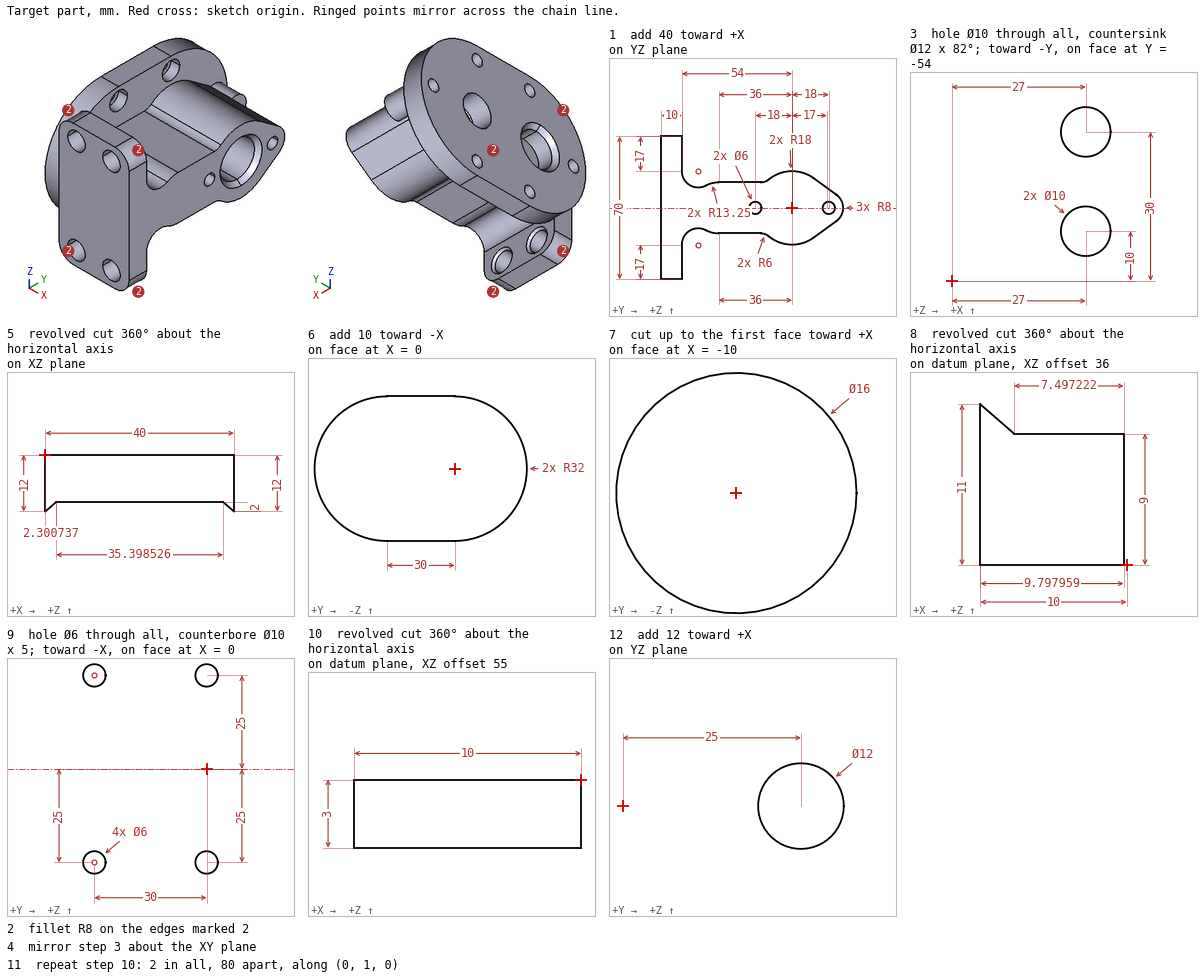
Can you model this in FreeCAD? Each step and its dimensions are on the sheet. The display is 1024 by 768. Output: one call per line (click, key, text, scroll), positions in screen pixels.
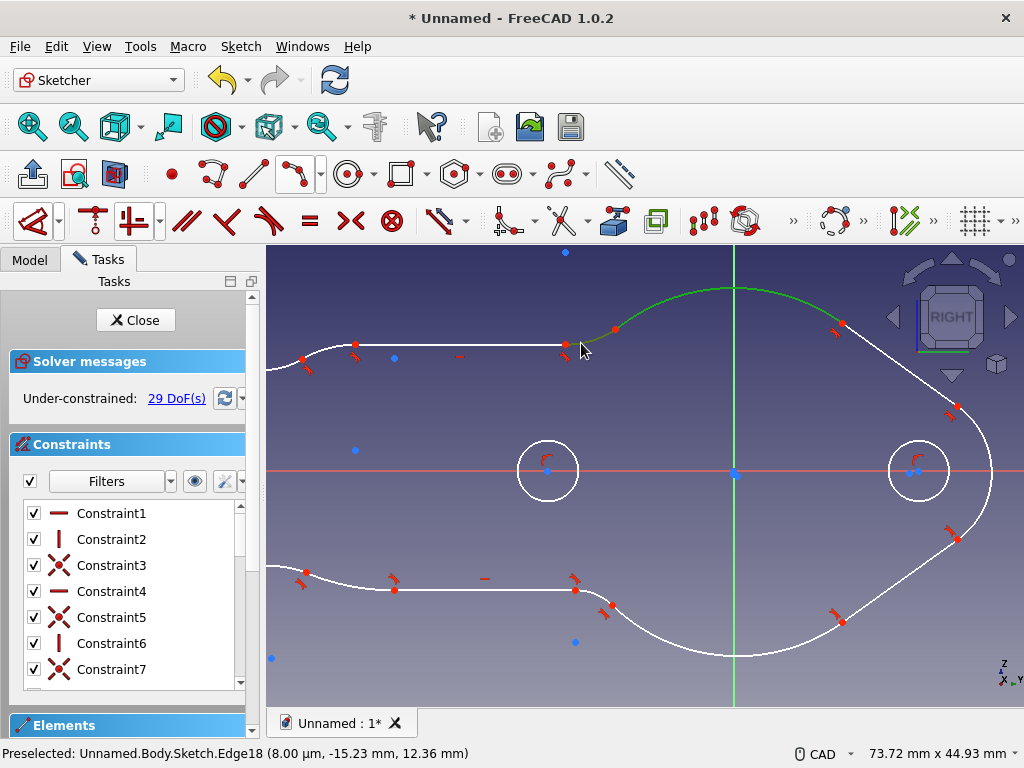
click(269, 222)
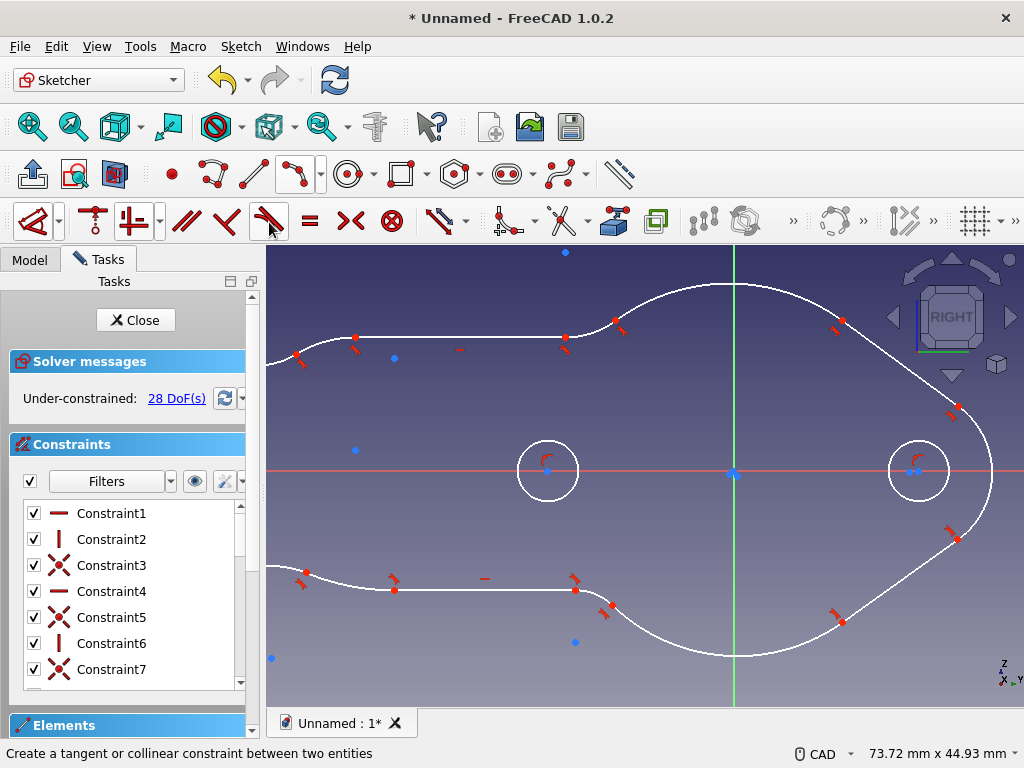
click(675, 645)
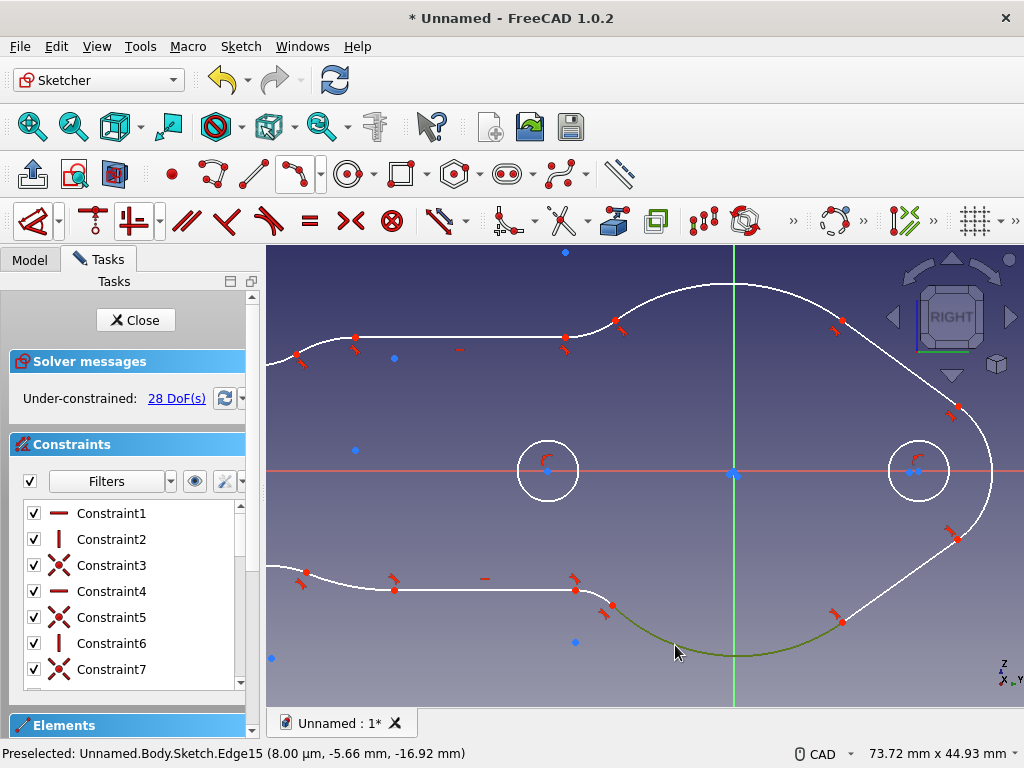
click(777, 290)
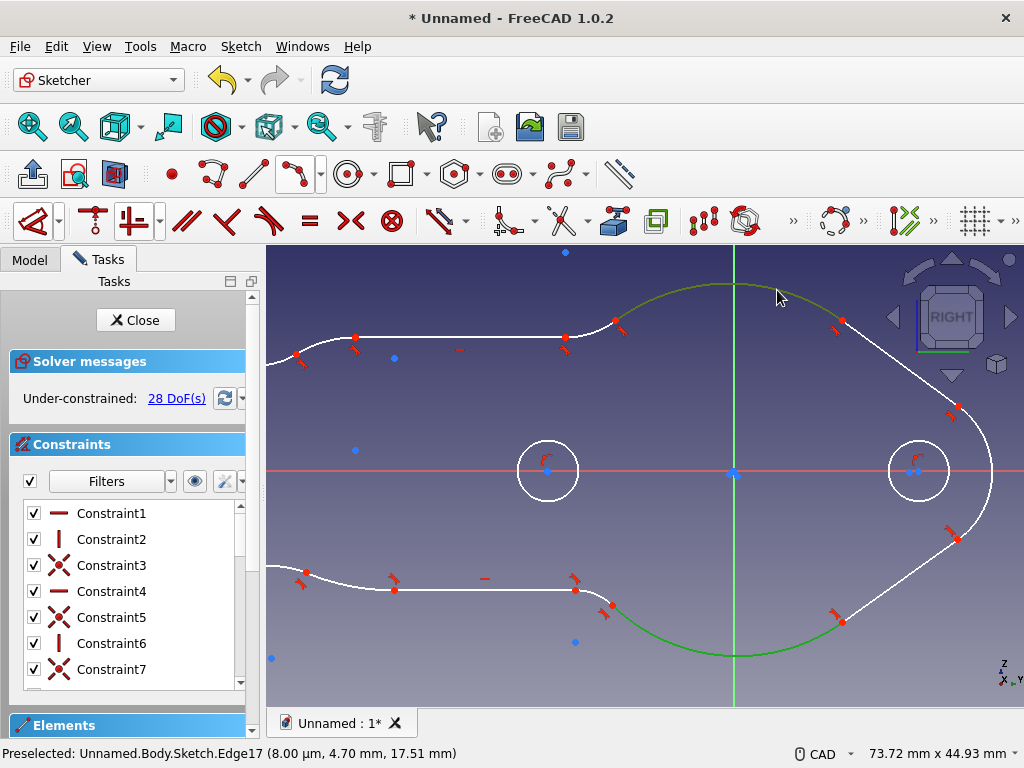
click(93, 222)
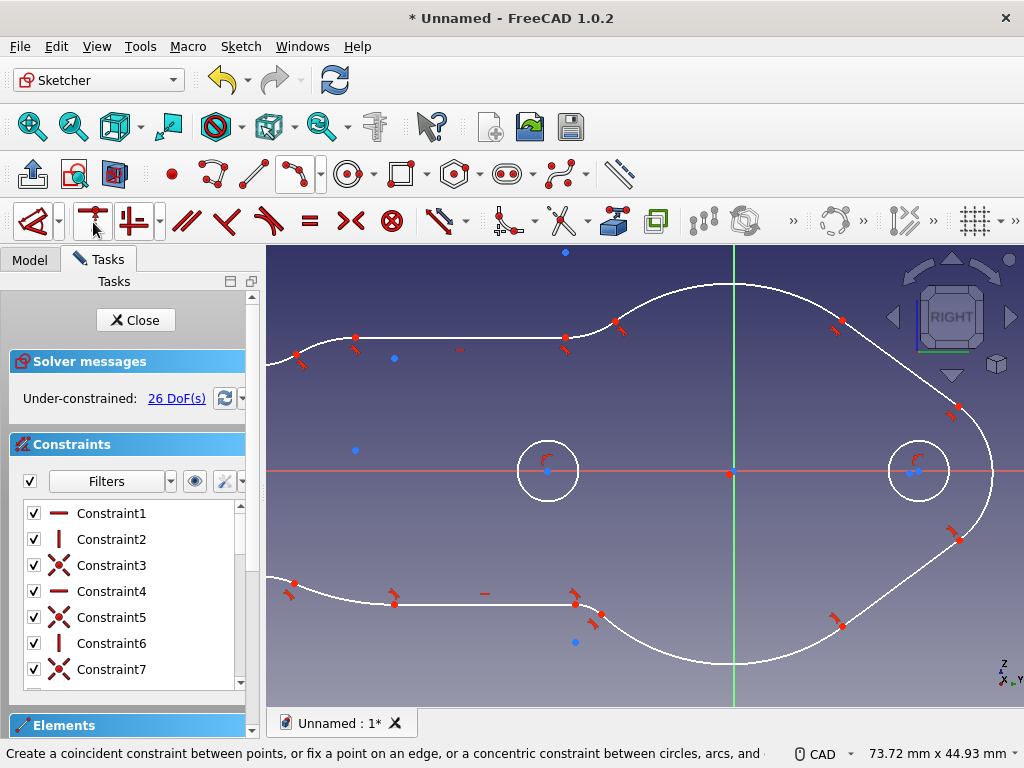
scroll(731, 473, up, 2)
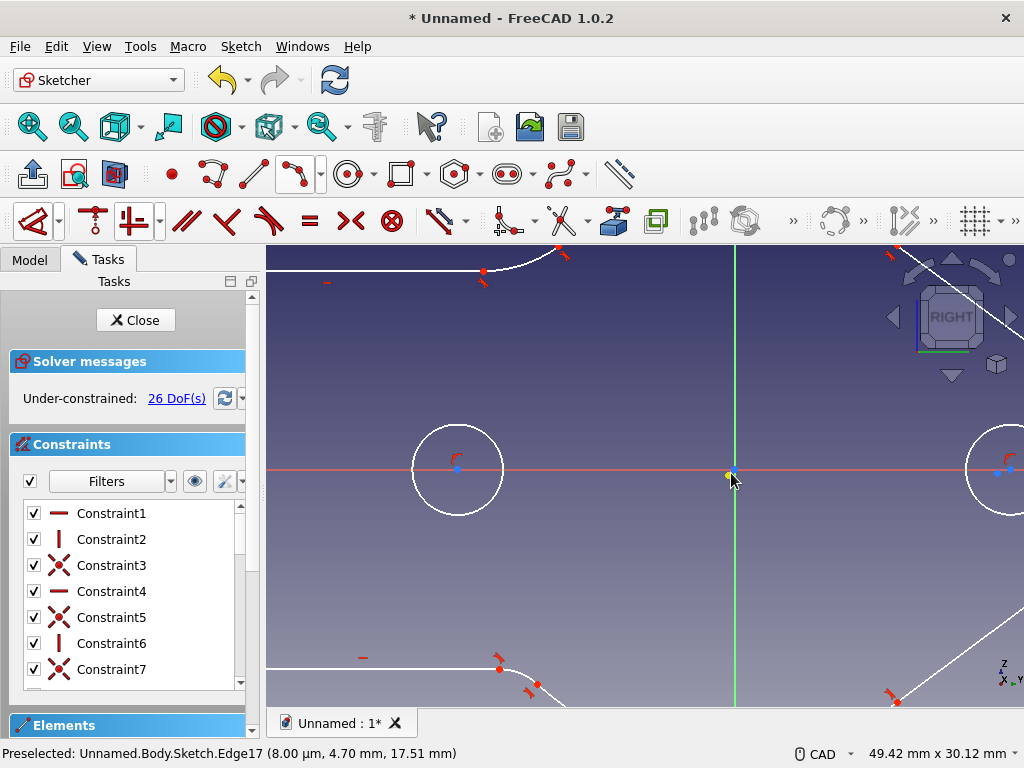
drag(718, 460, 745, 486)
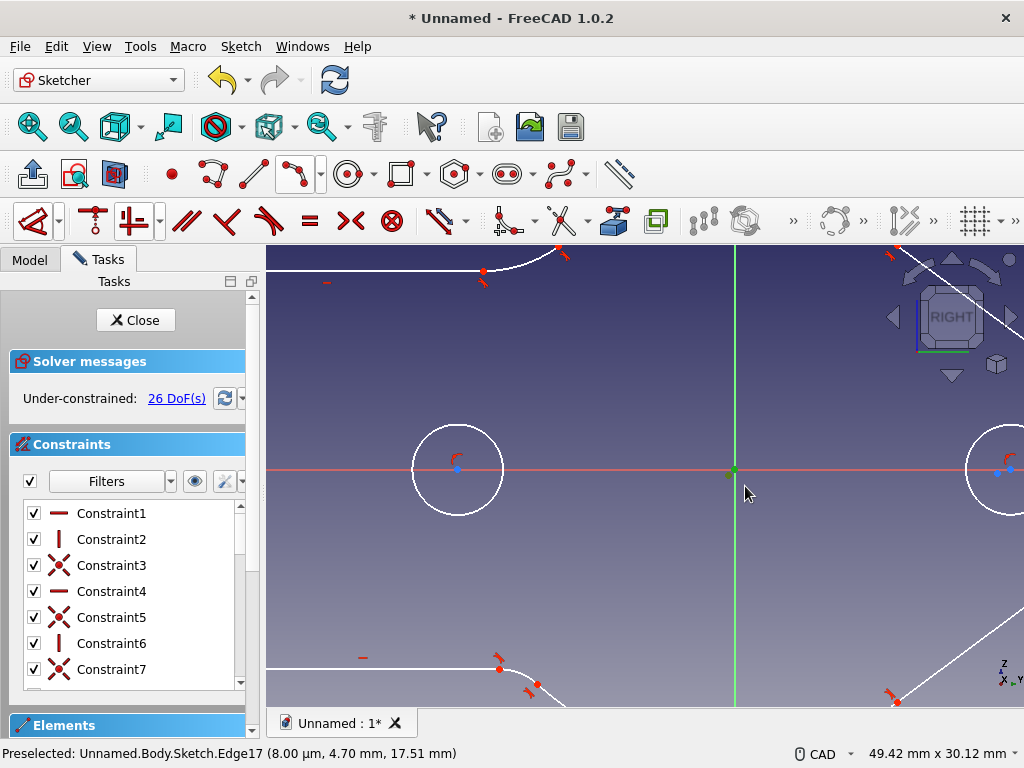
click(93, 222)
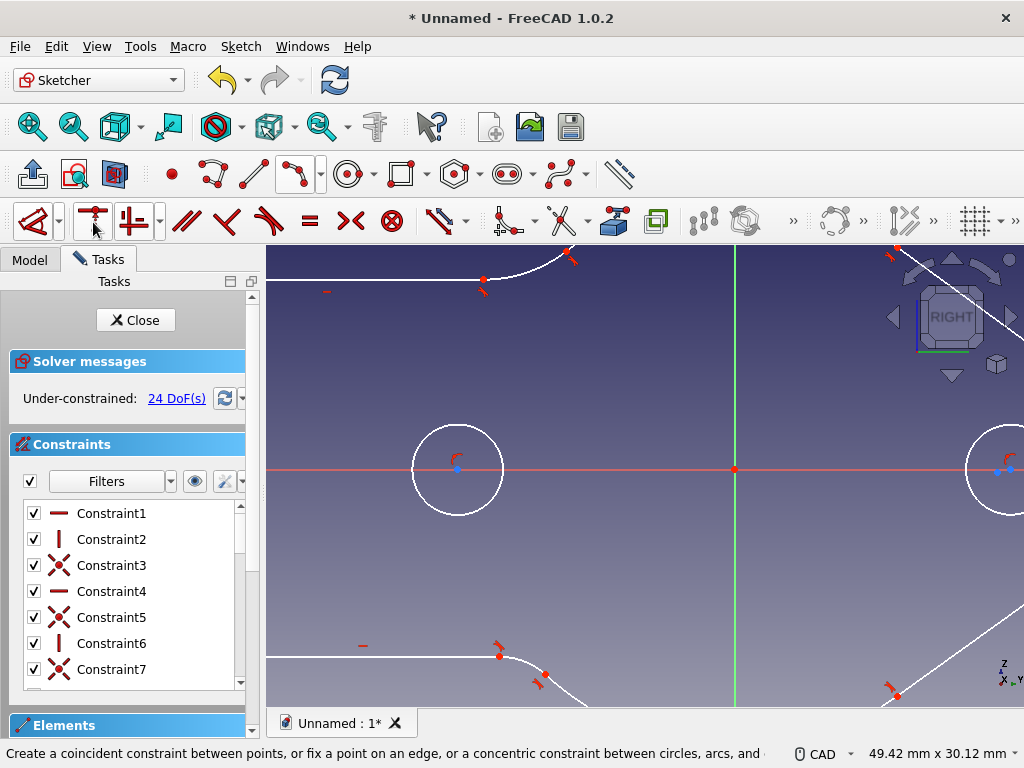
scroll(623, 478, down, 7)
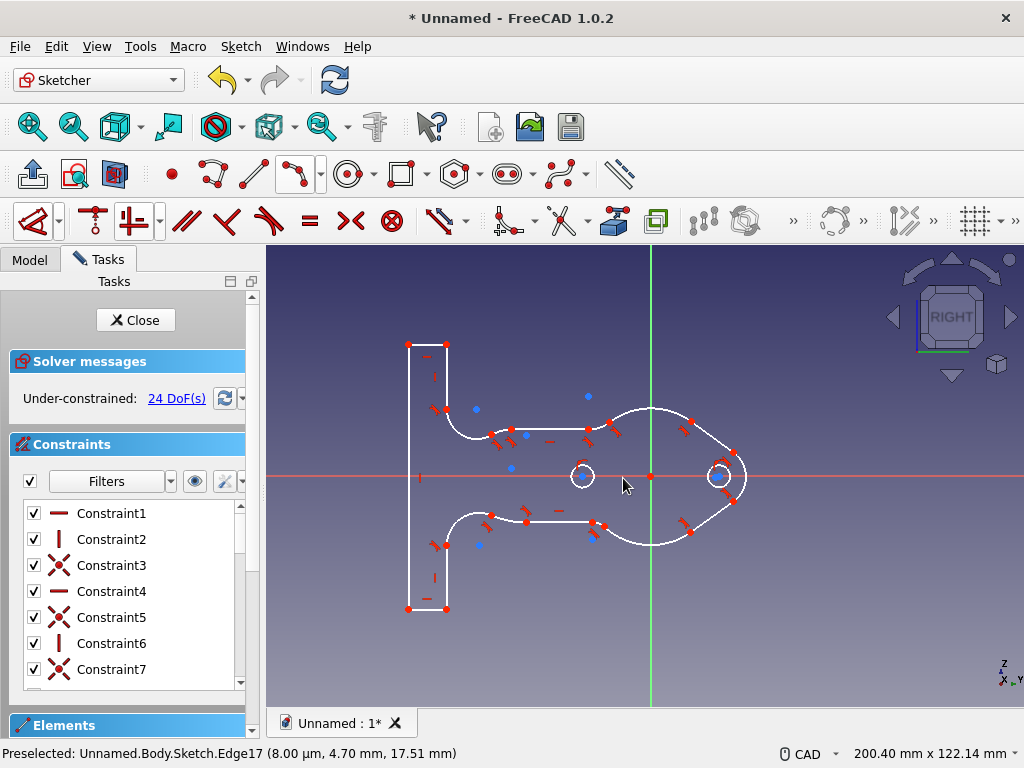
click(453, 427)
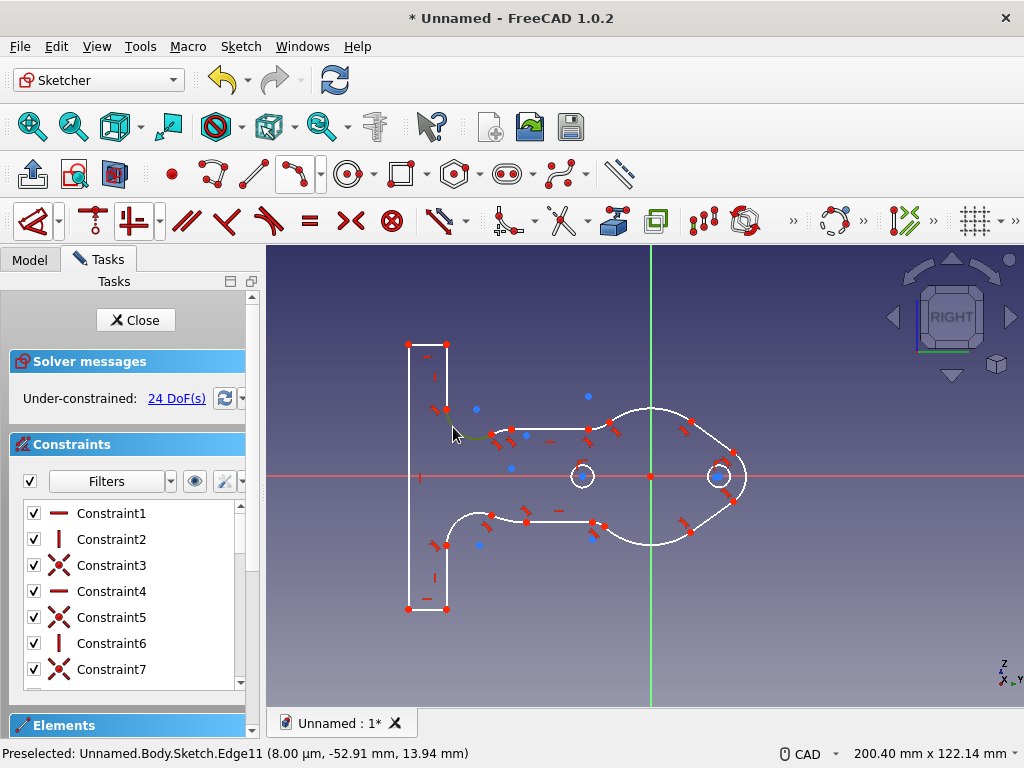
click(473, 513)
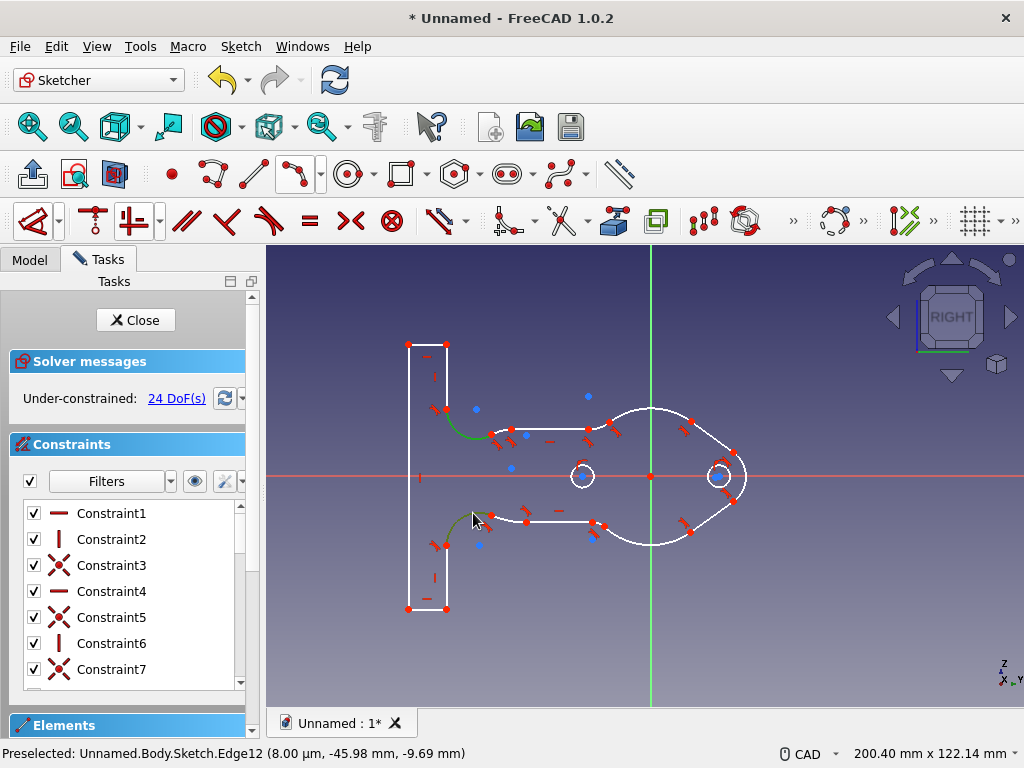
click(744, 488)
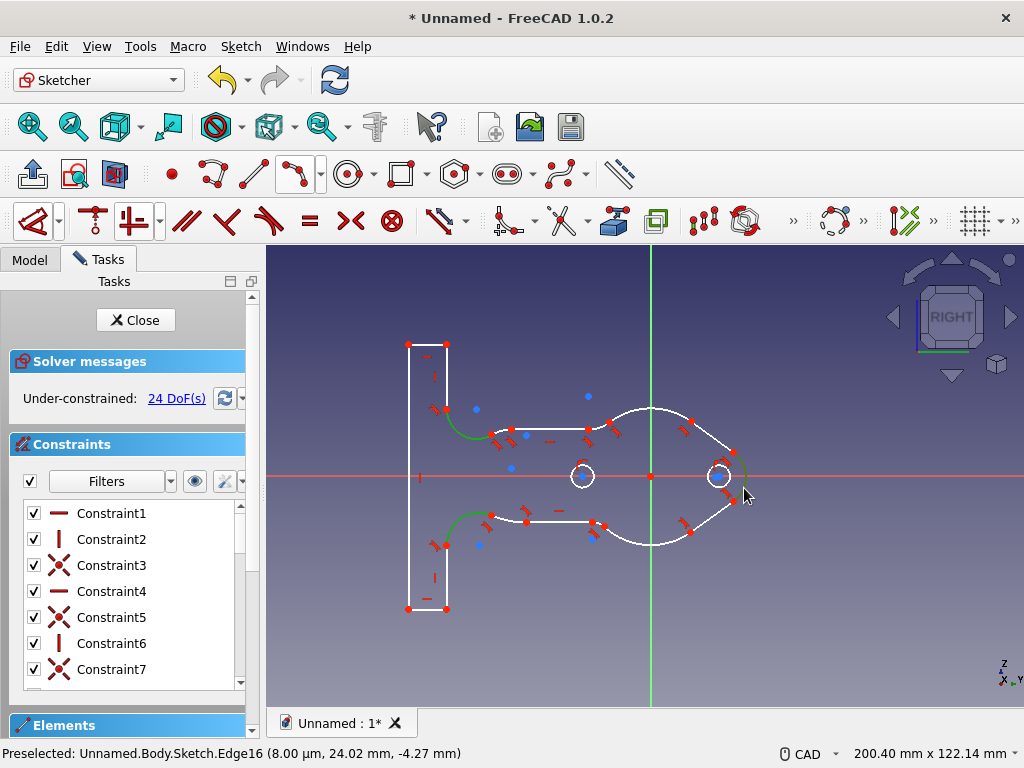
click(310, 222)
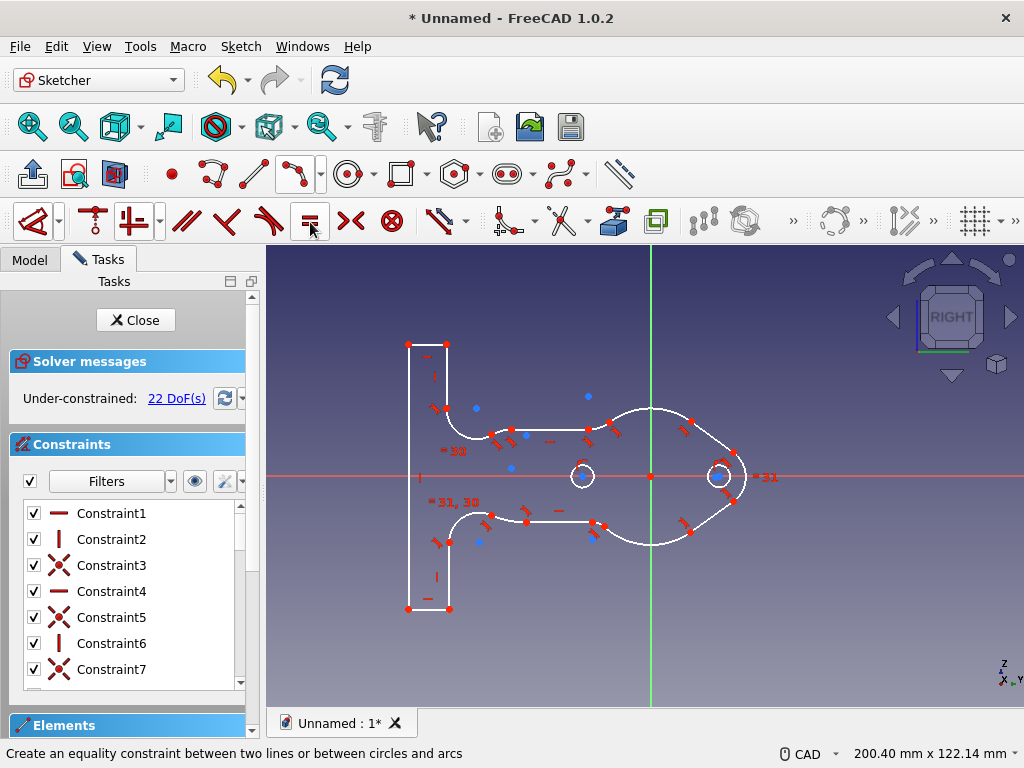
scroll(502, 431, up, 2)